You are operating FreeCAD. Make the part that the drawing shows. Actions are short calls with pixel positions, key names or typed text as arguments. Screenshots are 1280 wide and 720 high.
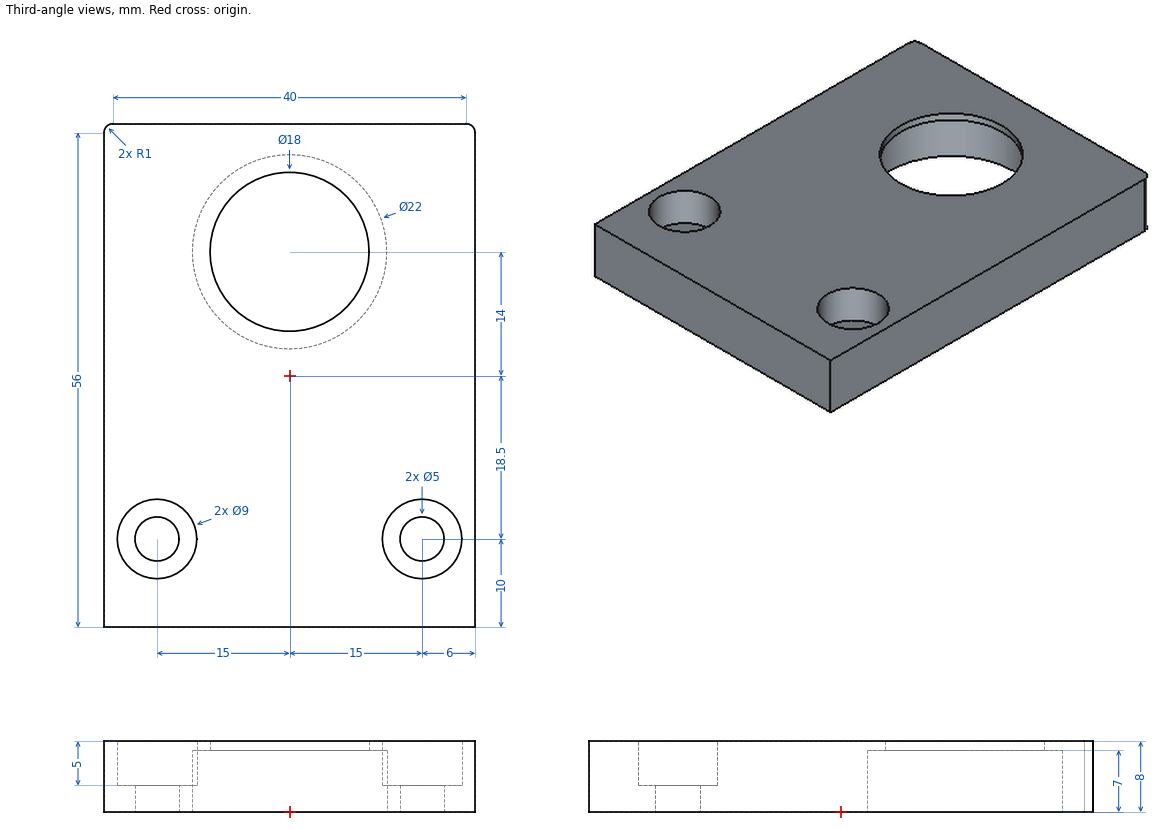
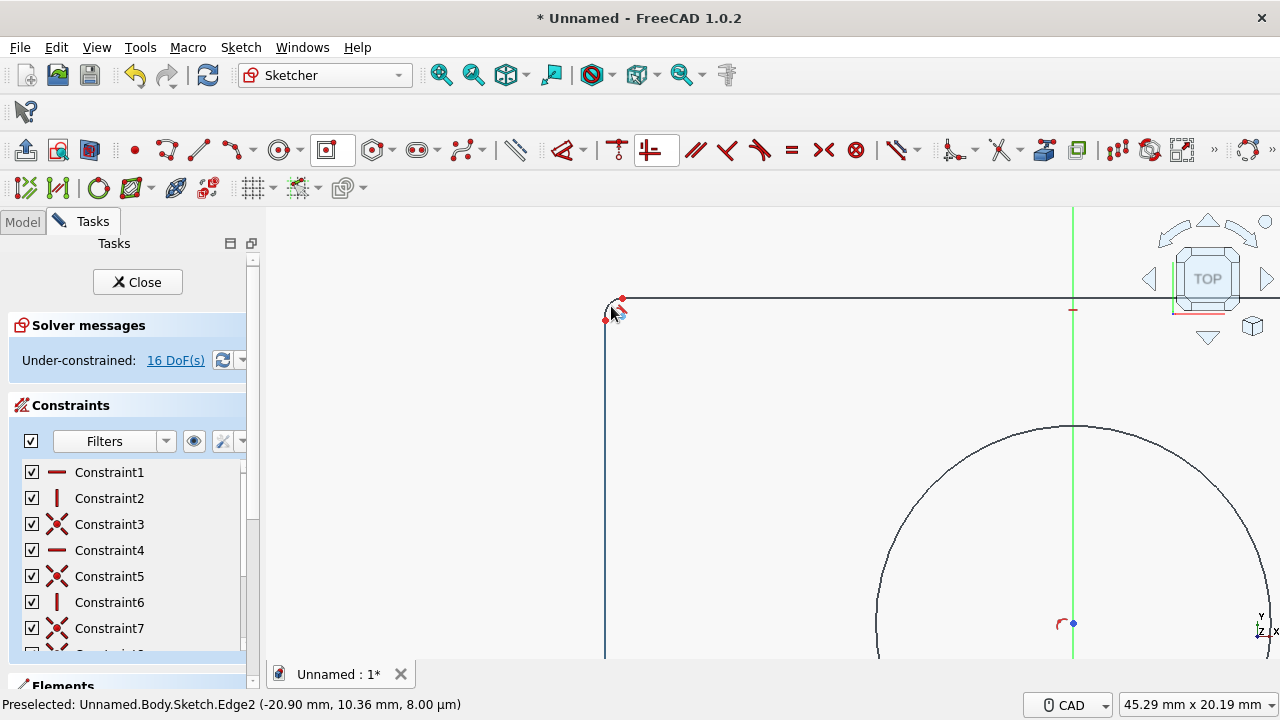
click(609, 305)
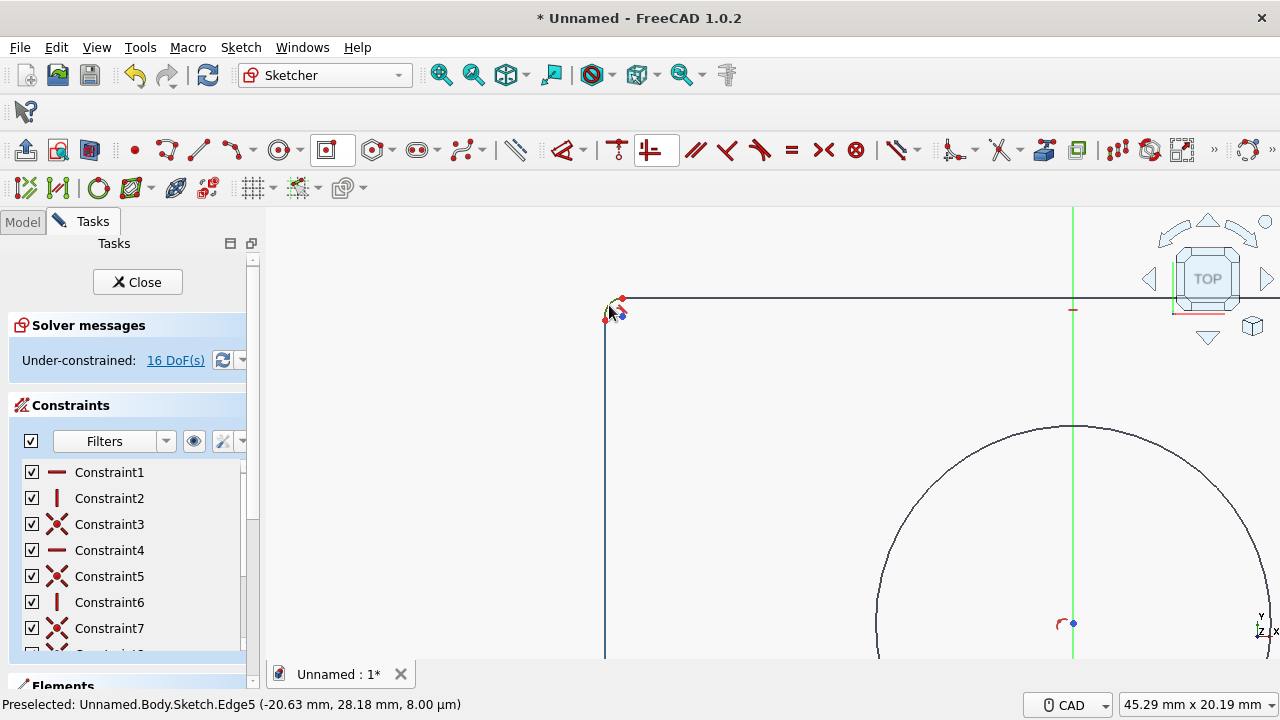
click(760, 150)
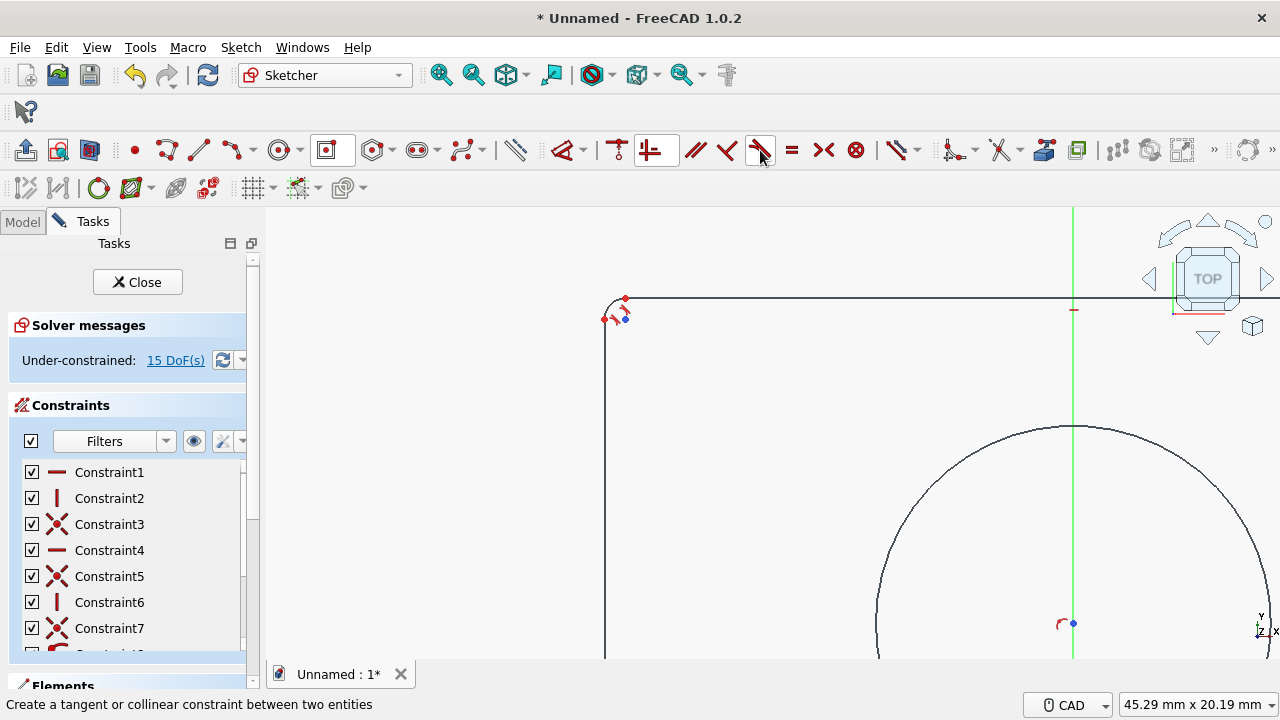
scroll(611, 306, down, 8)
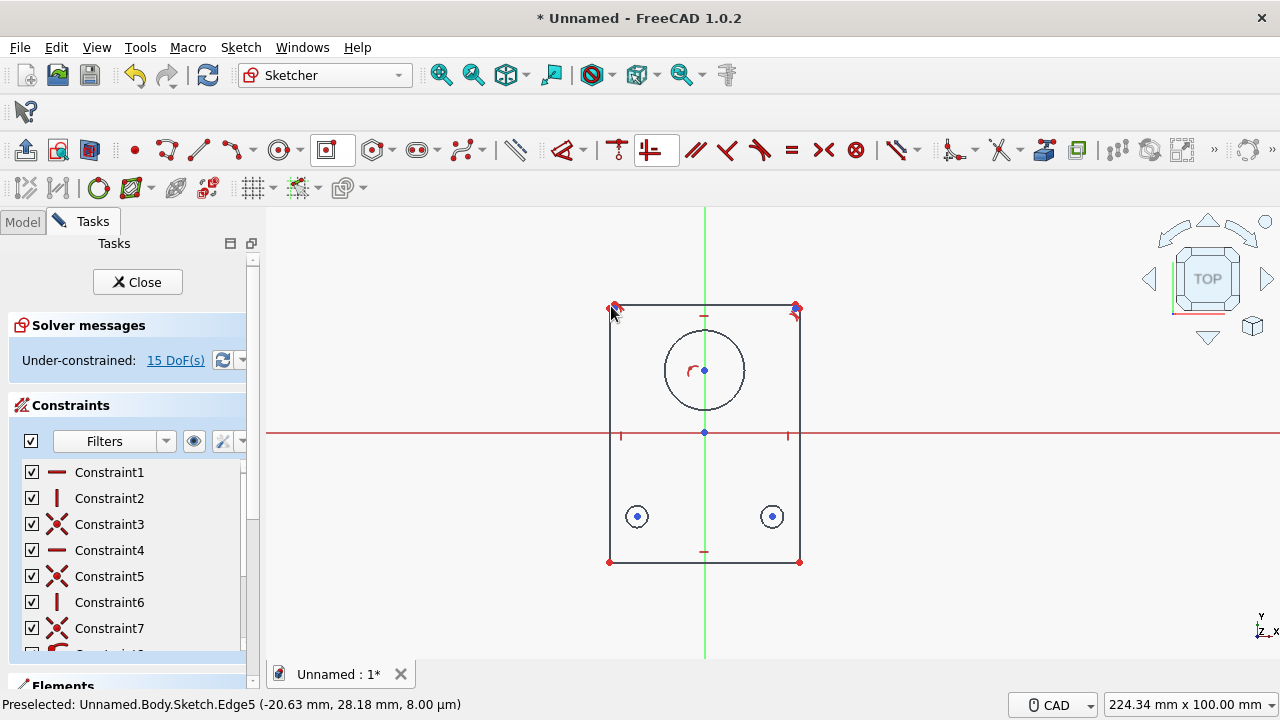
click(800, 487)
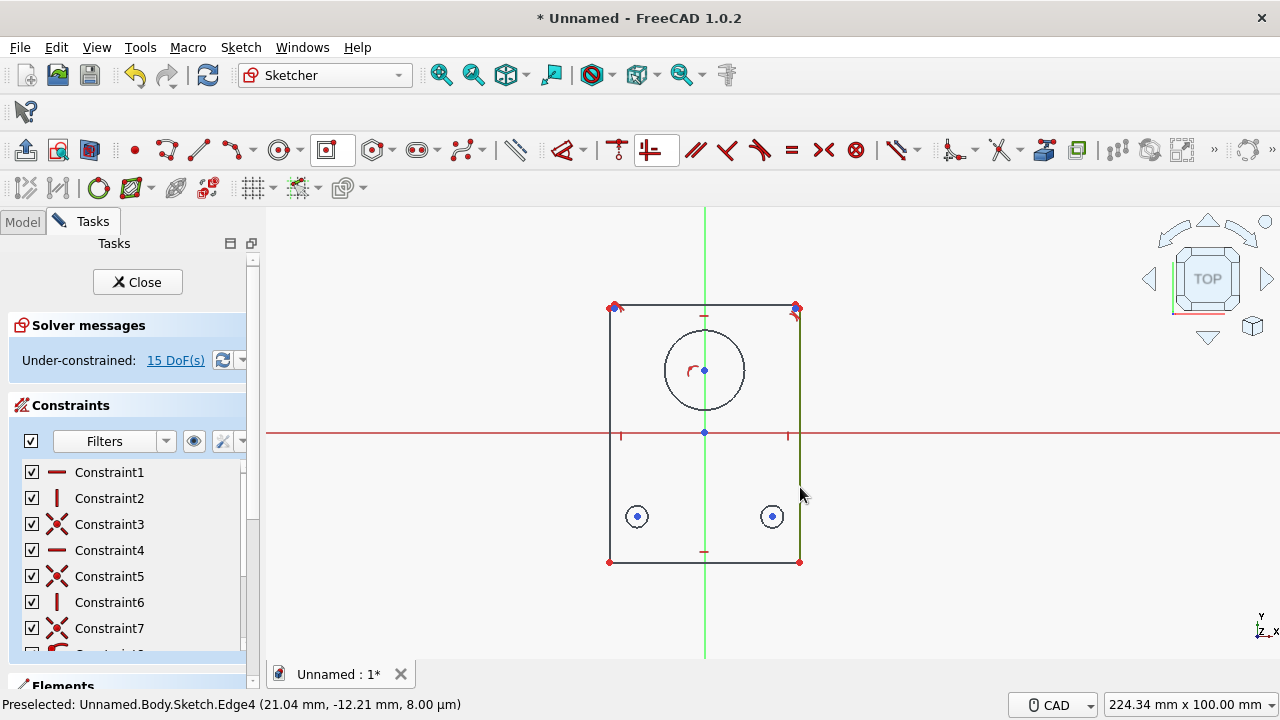
scroll(799, 306, up, 8)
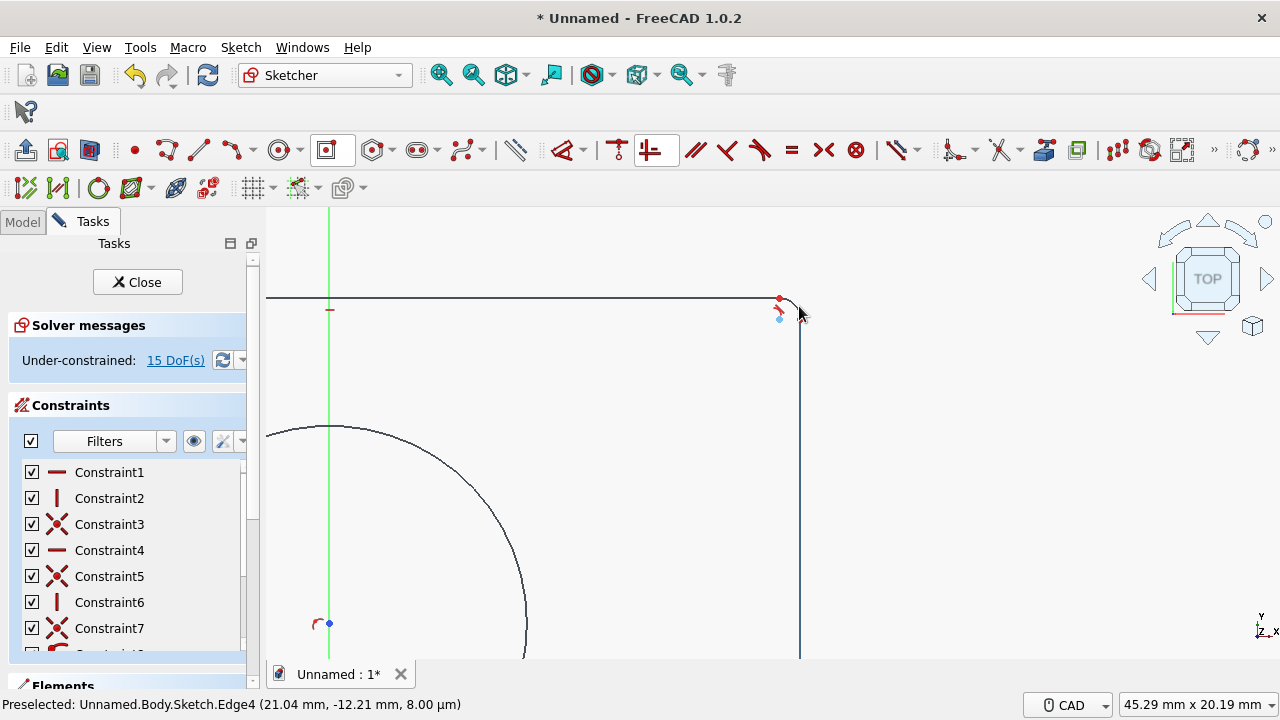
click(795, 305)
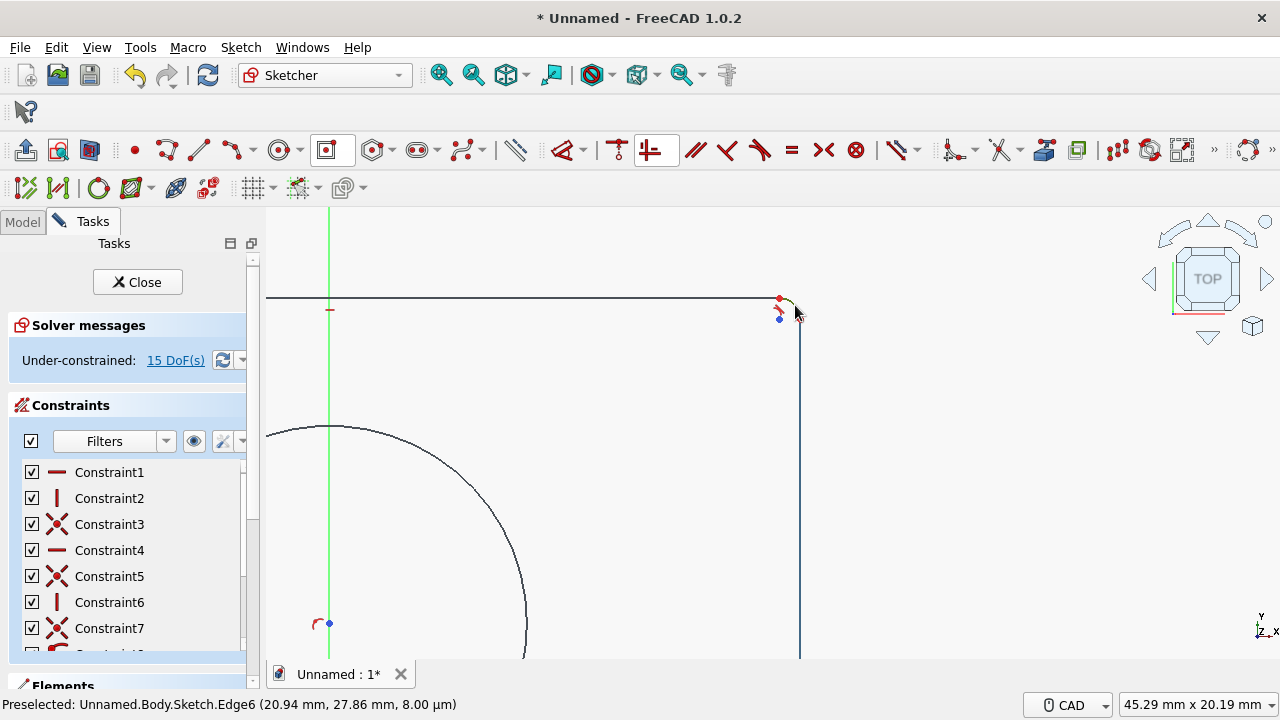
click(760, 150)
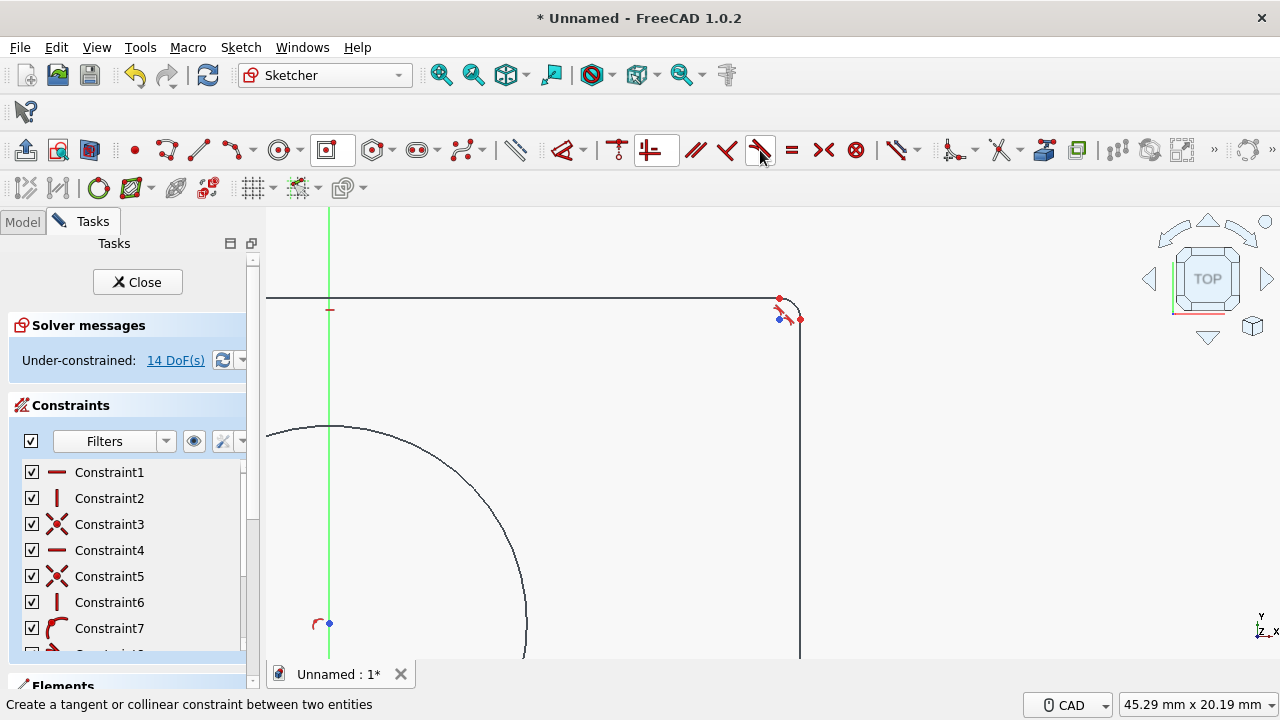
scroll(799, 306, down, 8)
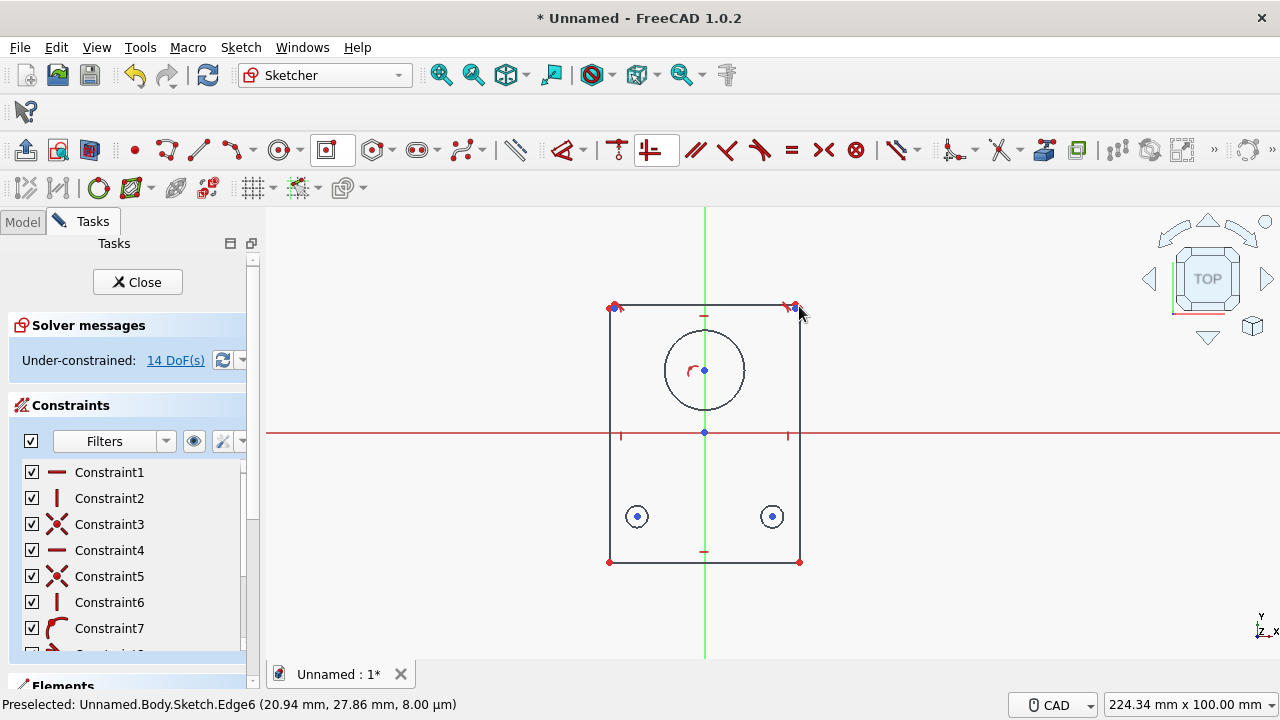
scroll(612, 305, up, 10)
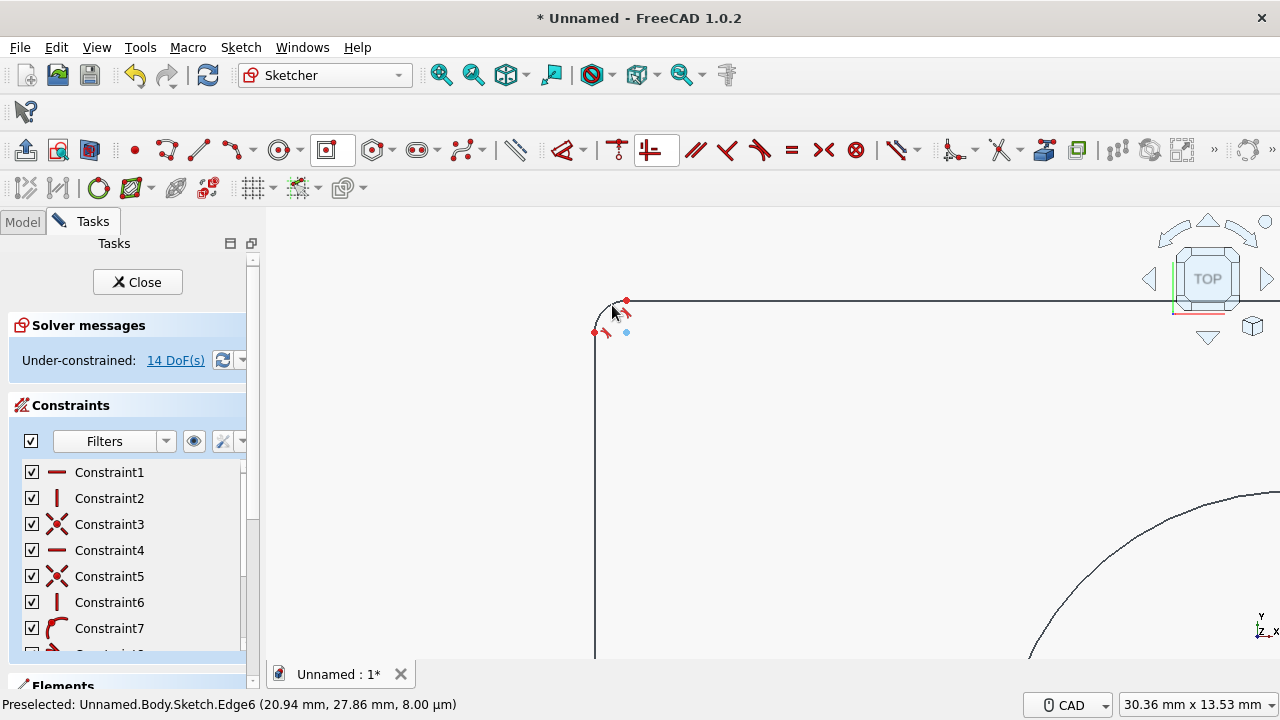
click(612, 304)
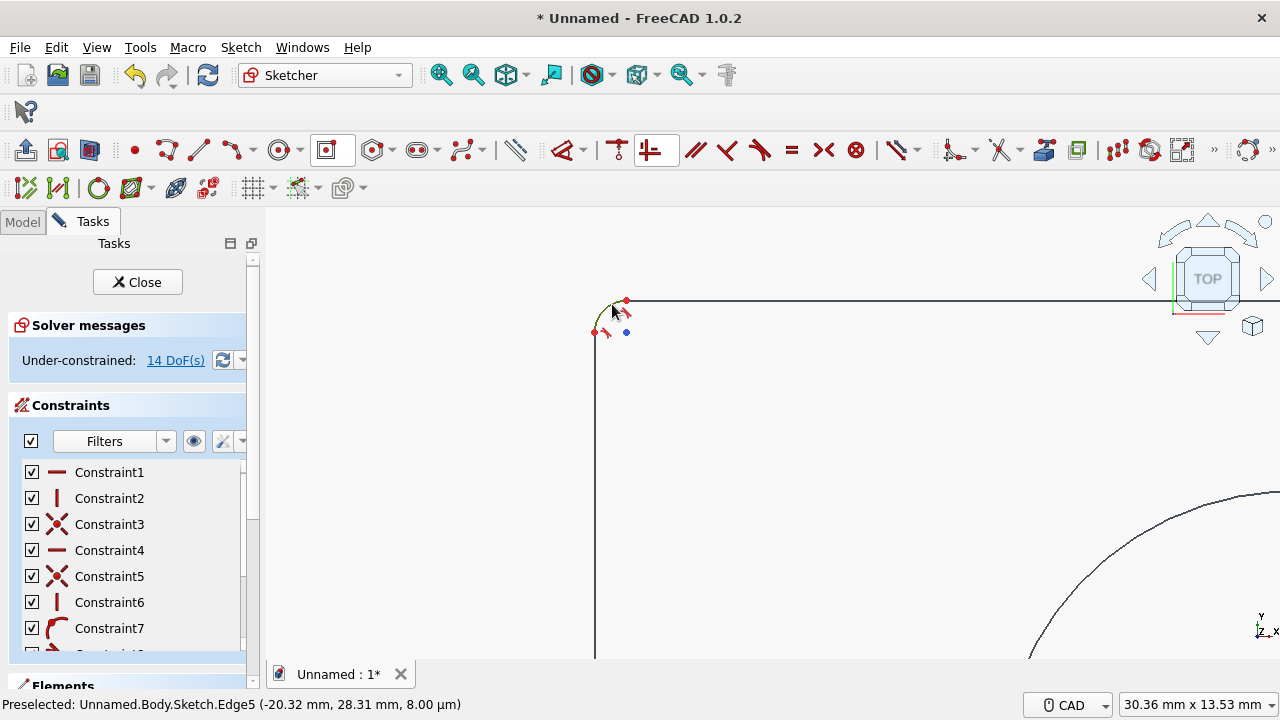
scroll(612, 305, down, 10)